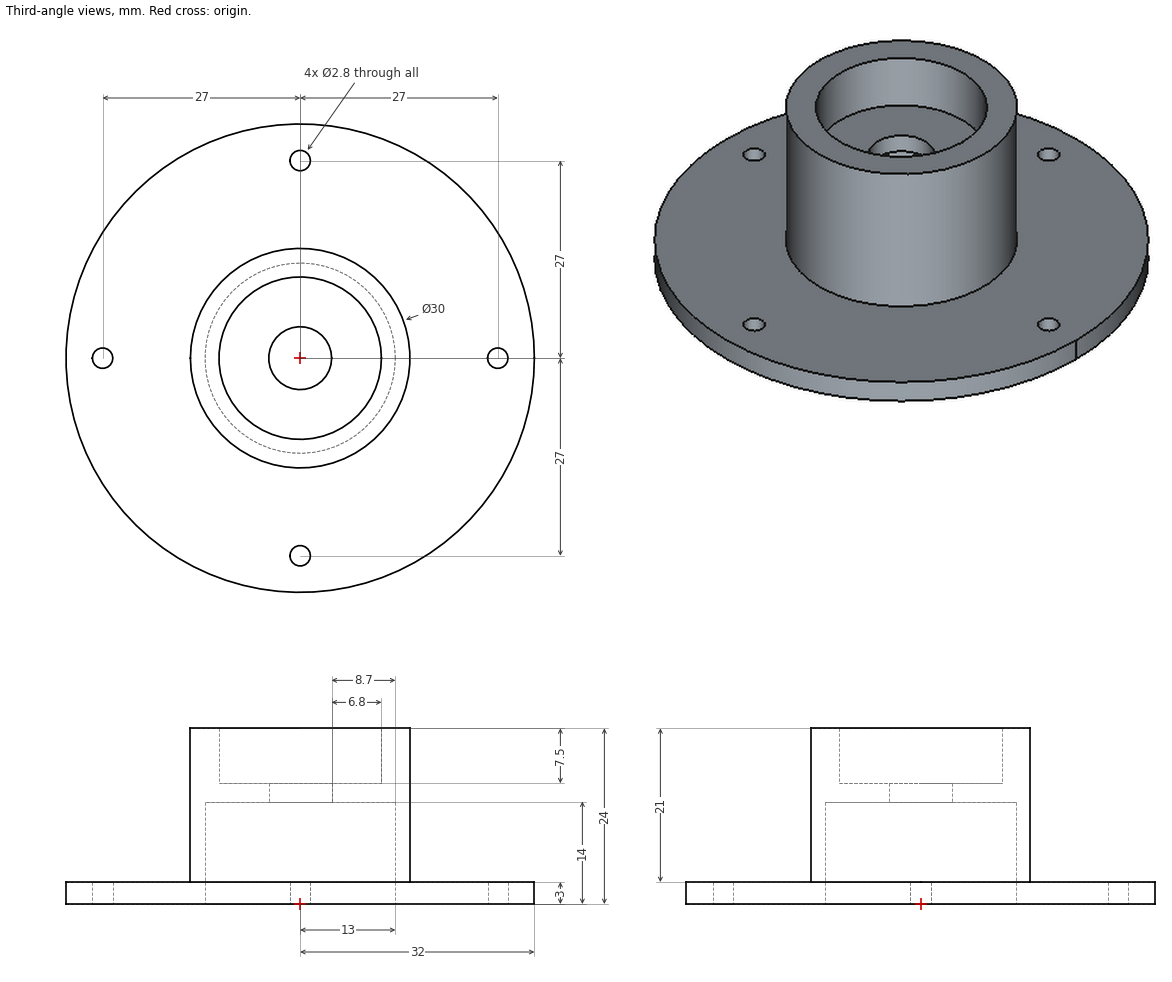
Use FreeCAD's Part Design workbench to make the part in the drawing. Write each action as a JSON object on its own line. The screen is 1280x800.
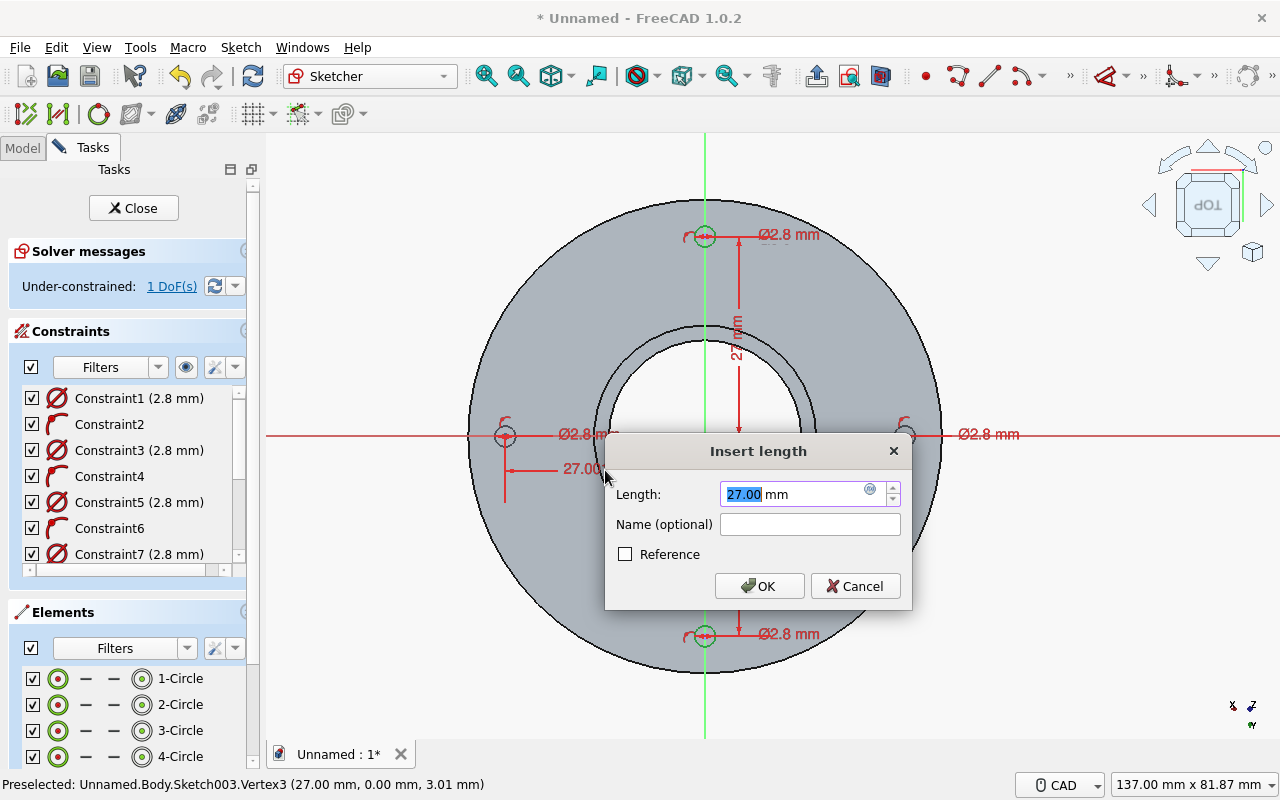
{"action": "type", "text": "27"}
{"action": "key", "text": "Return"}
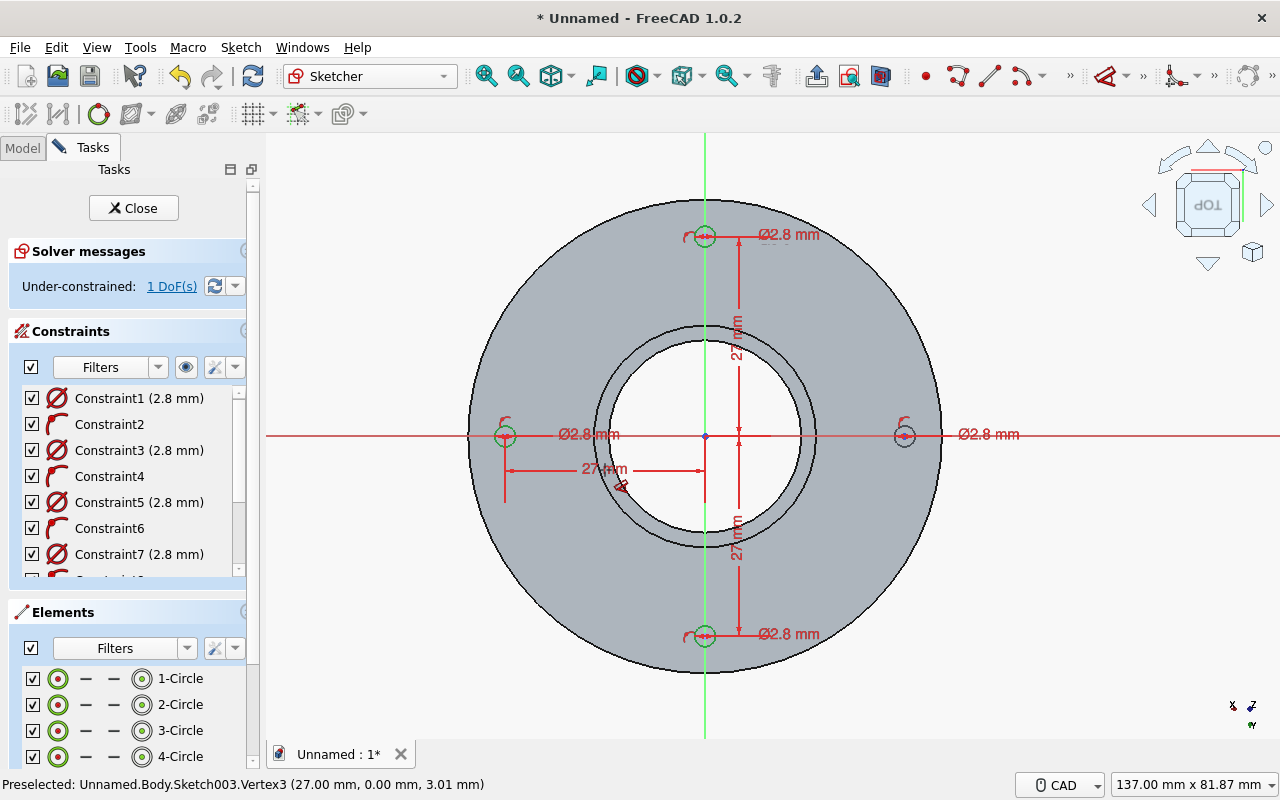
{"action": "left_click", "coordinate": [905, 436]}
{"action": "left_click", "coordinate": [805, 470]}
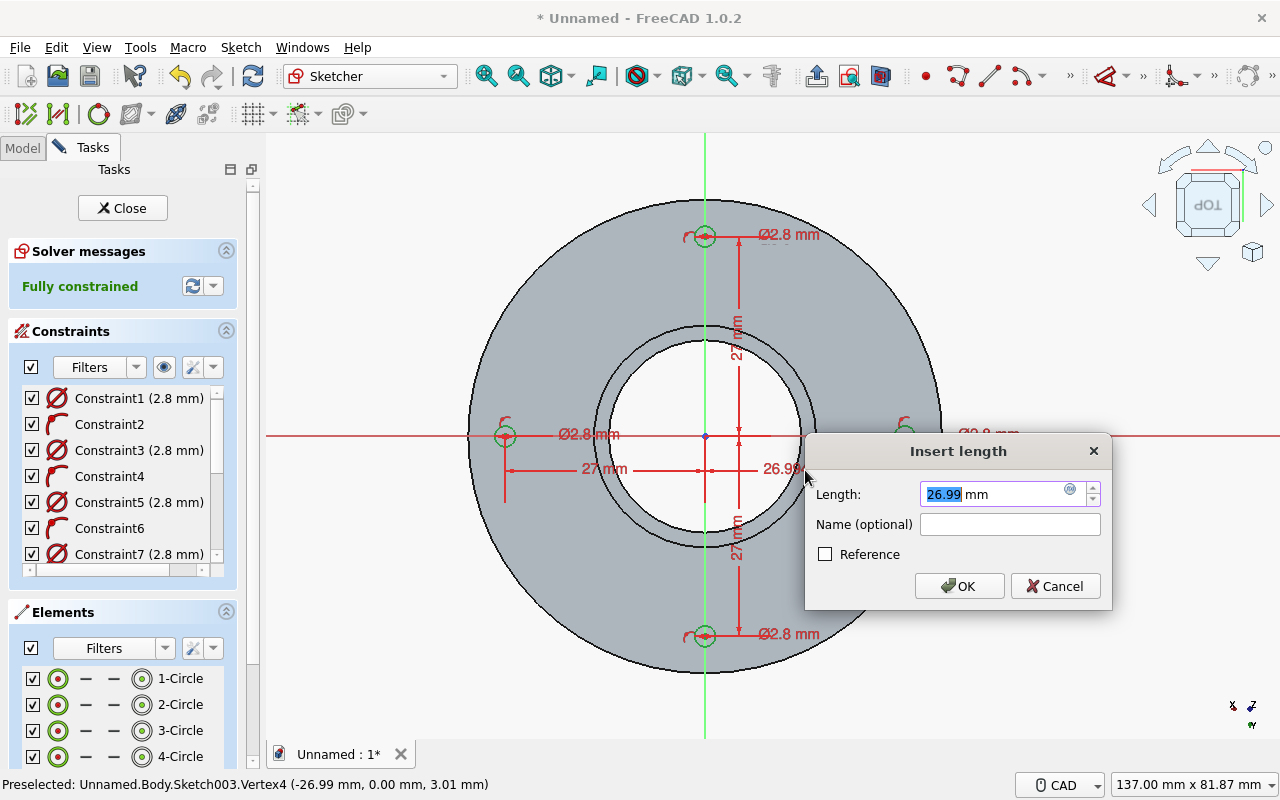
{"action": "type", "text": "27"}
{"action": "key", "text": "Return"}
{"action": "key", "text": "Escape"}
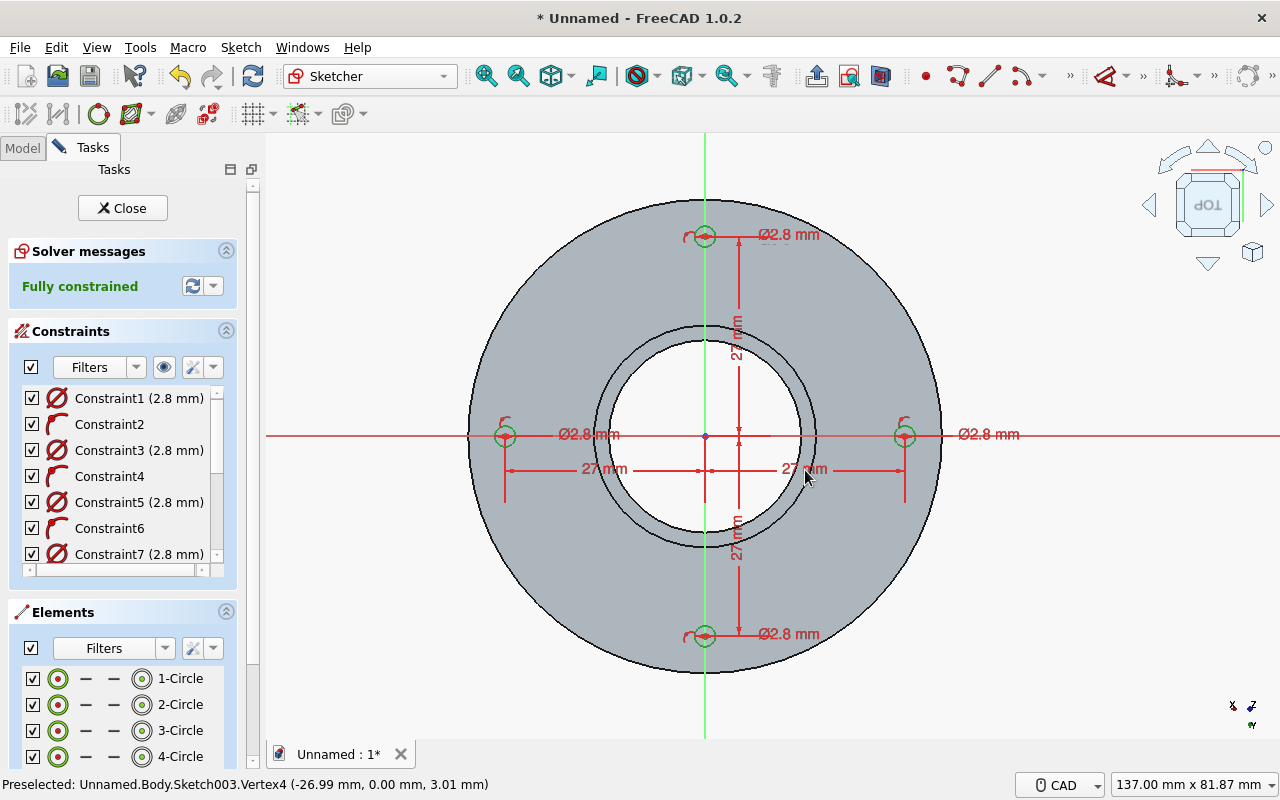
{"action": "left_click", "coordinate": [123, 208]}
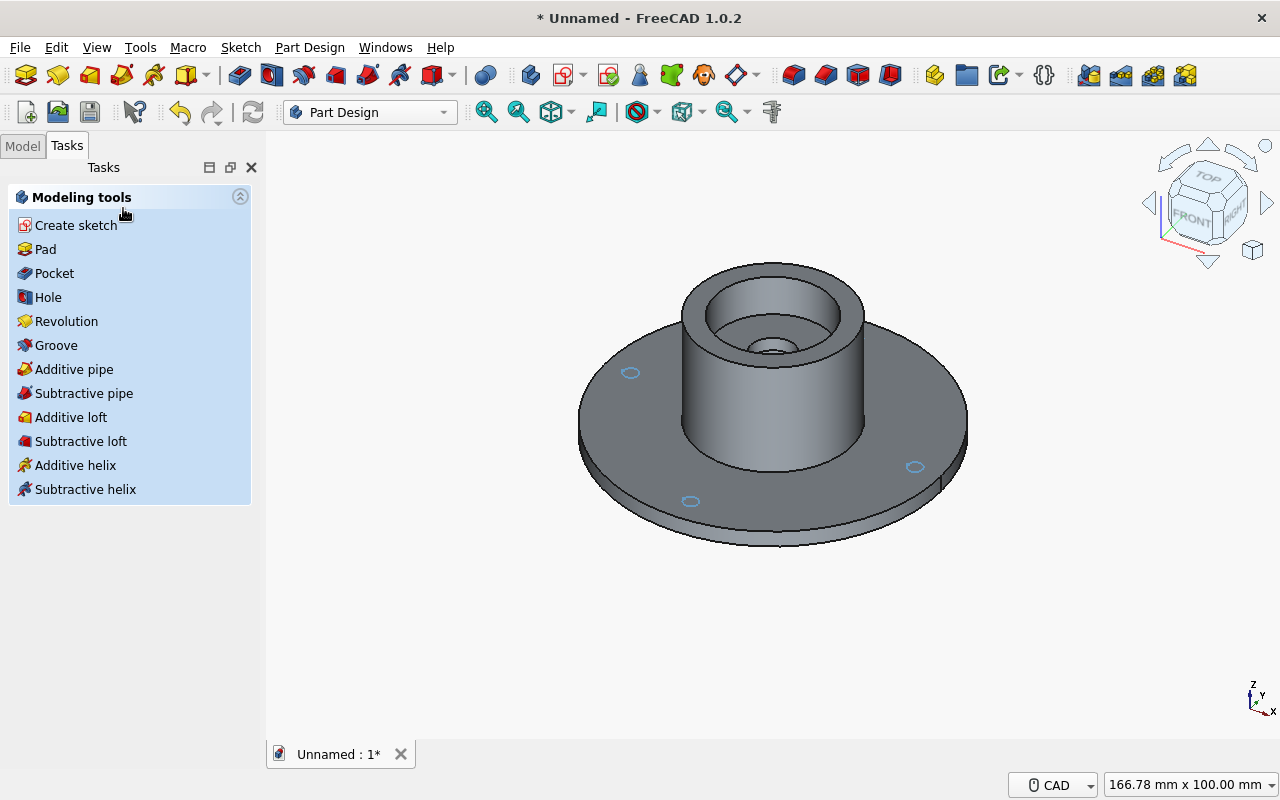
{"action": "left_click", "coordinate": [272, 76]}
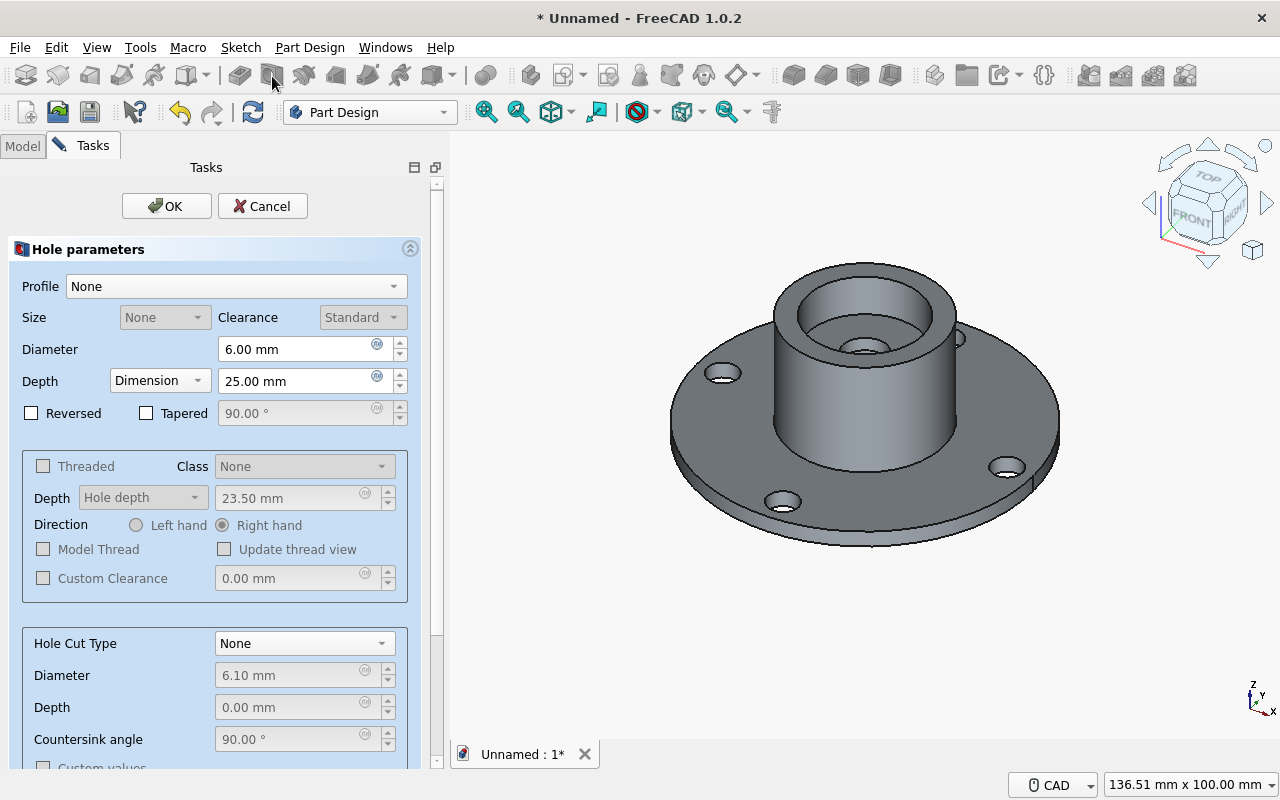
{"action": "triple_click", "coordinate": [305, 349]}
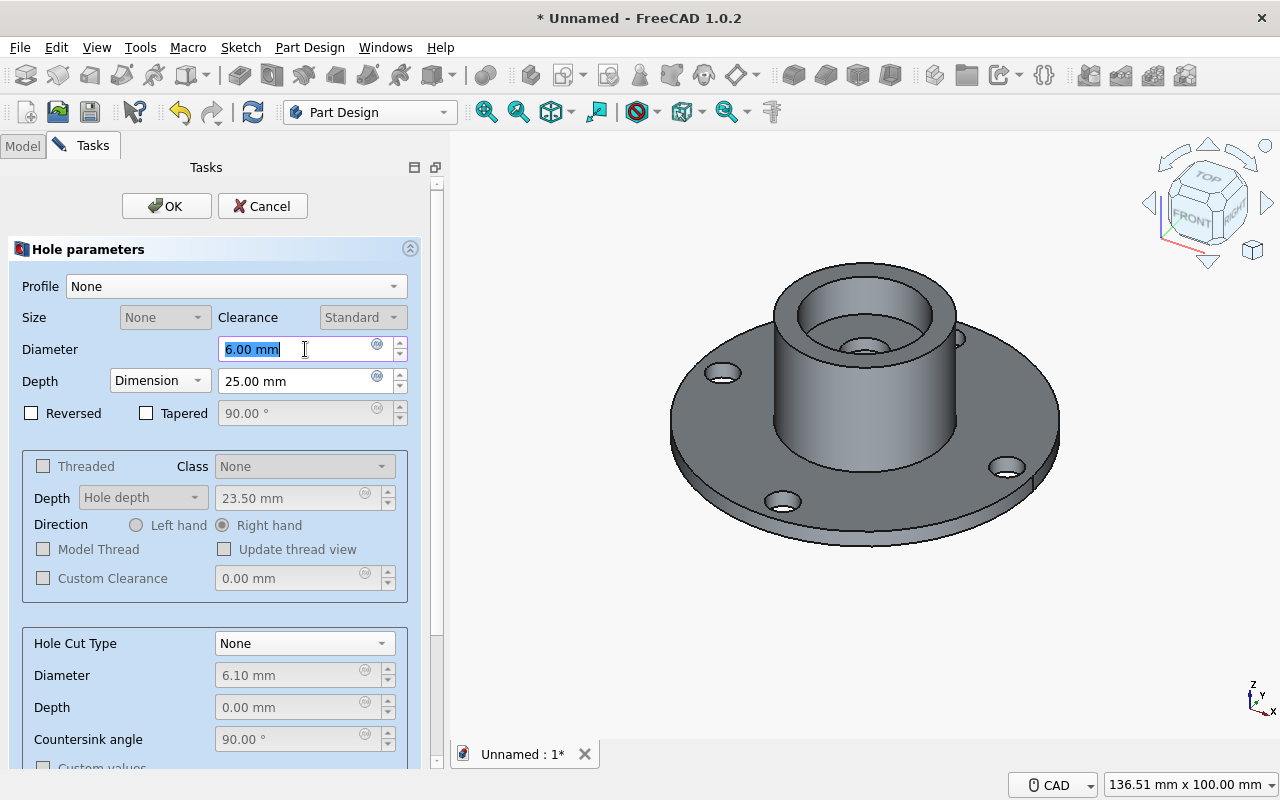
{"action": "type", "text": "2.8"}
{"action": "key", "text": "Tab"}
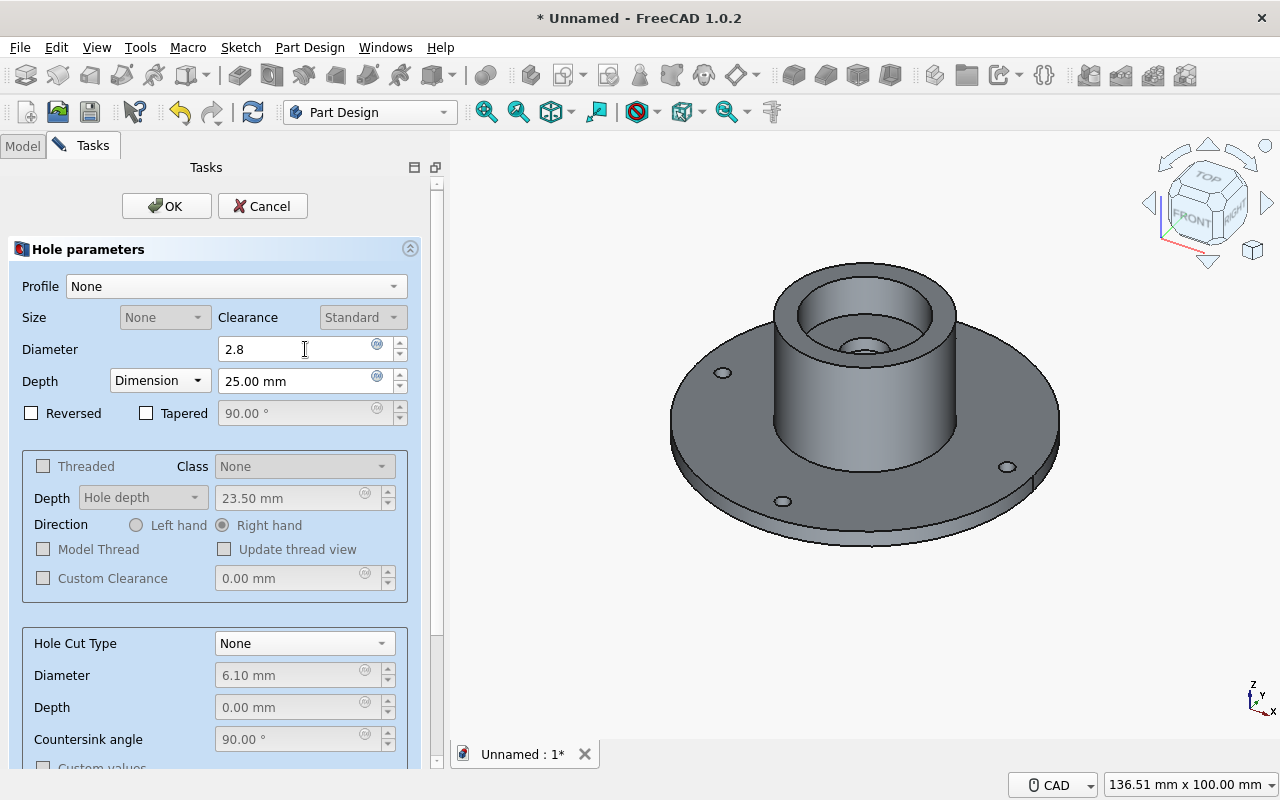
{"action": "left_click", "coordinate": [161, 380]}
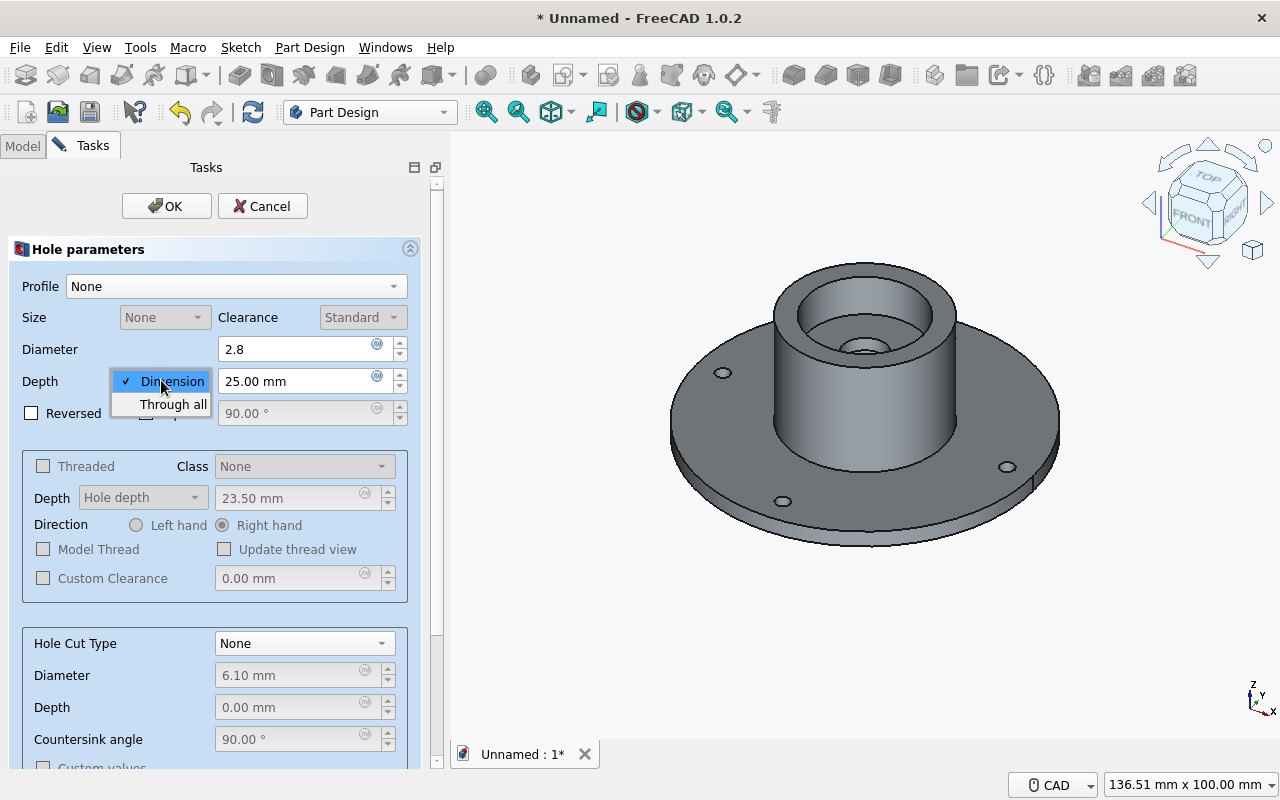
{"action": "left_click", "coordinate": [160, 404]}